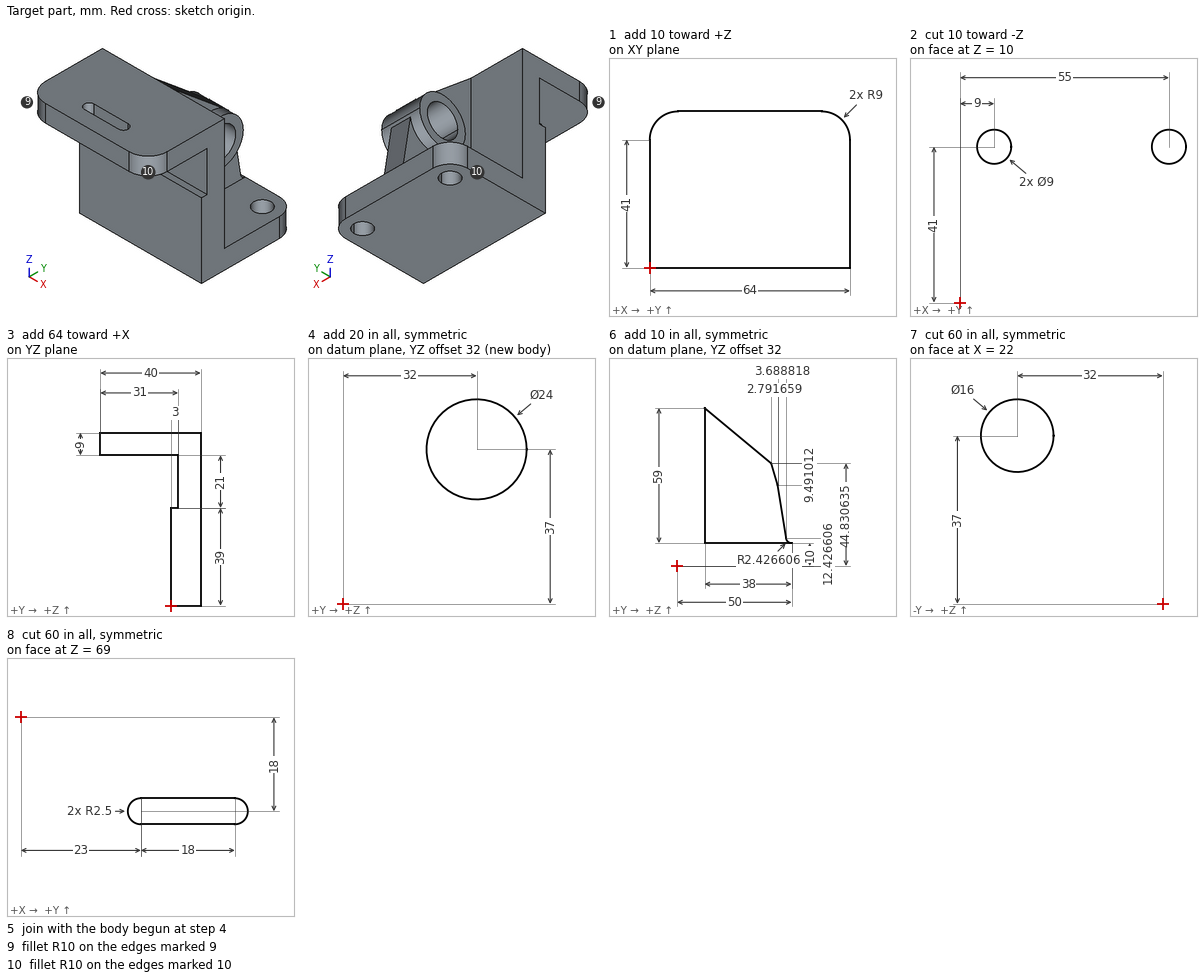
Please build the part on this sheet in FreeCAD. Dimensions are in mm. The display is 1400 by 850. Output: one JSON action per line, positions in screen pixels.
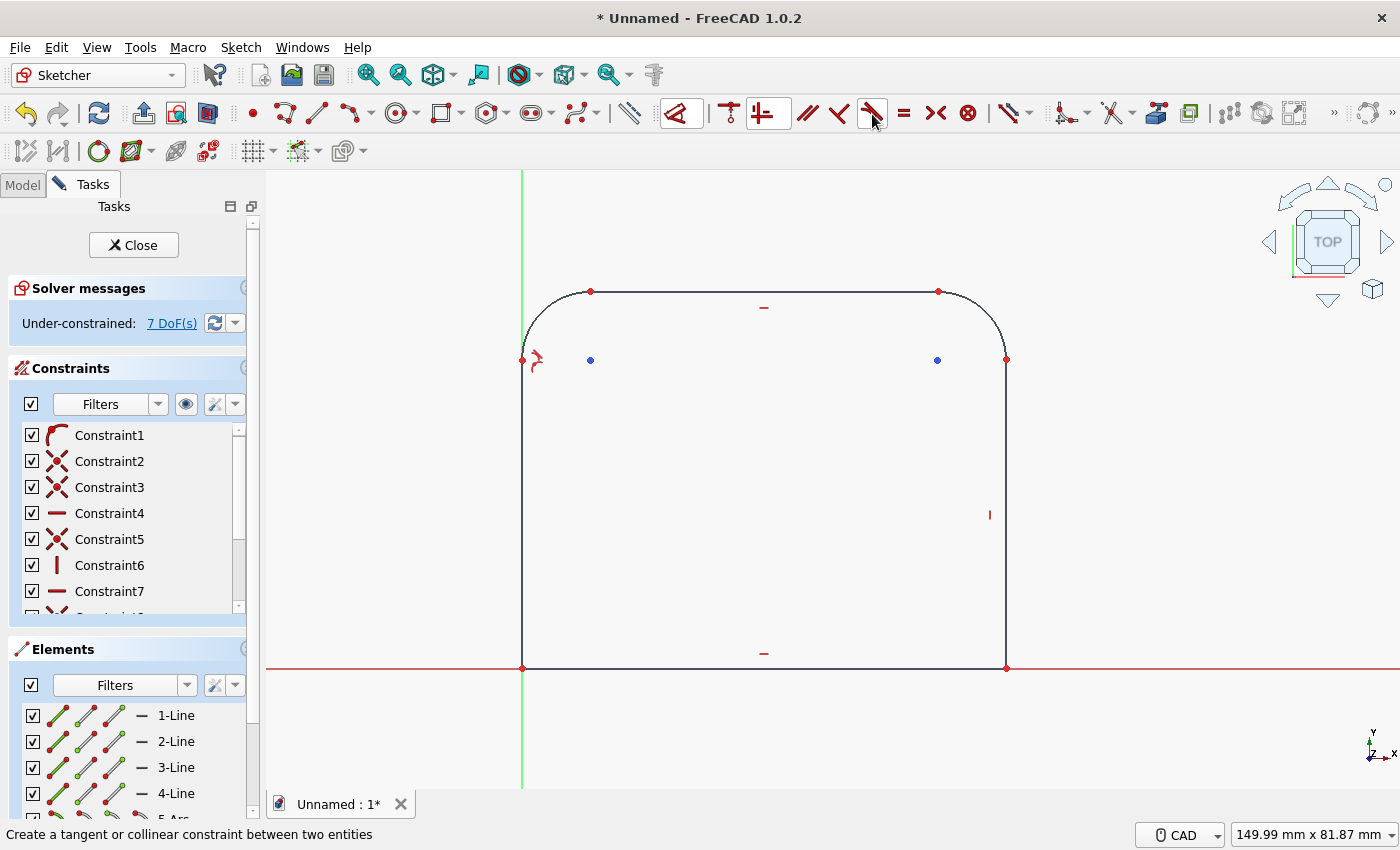
{"action": "left_click", "coordinate": [1006, 576]}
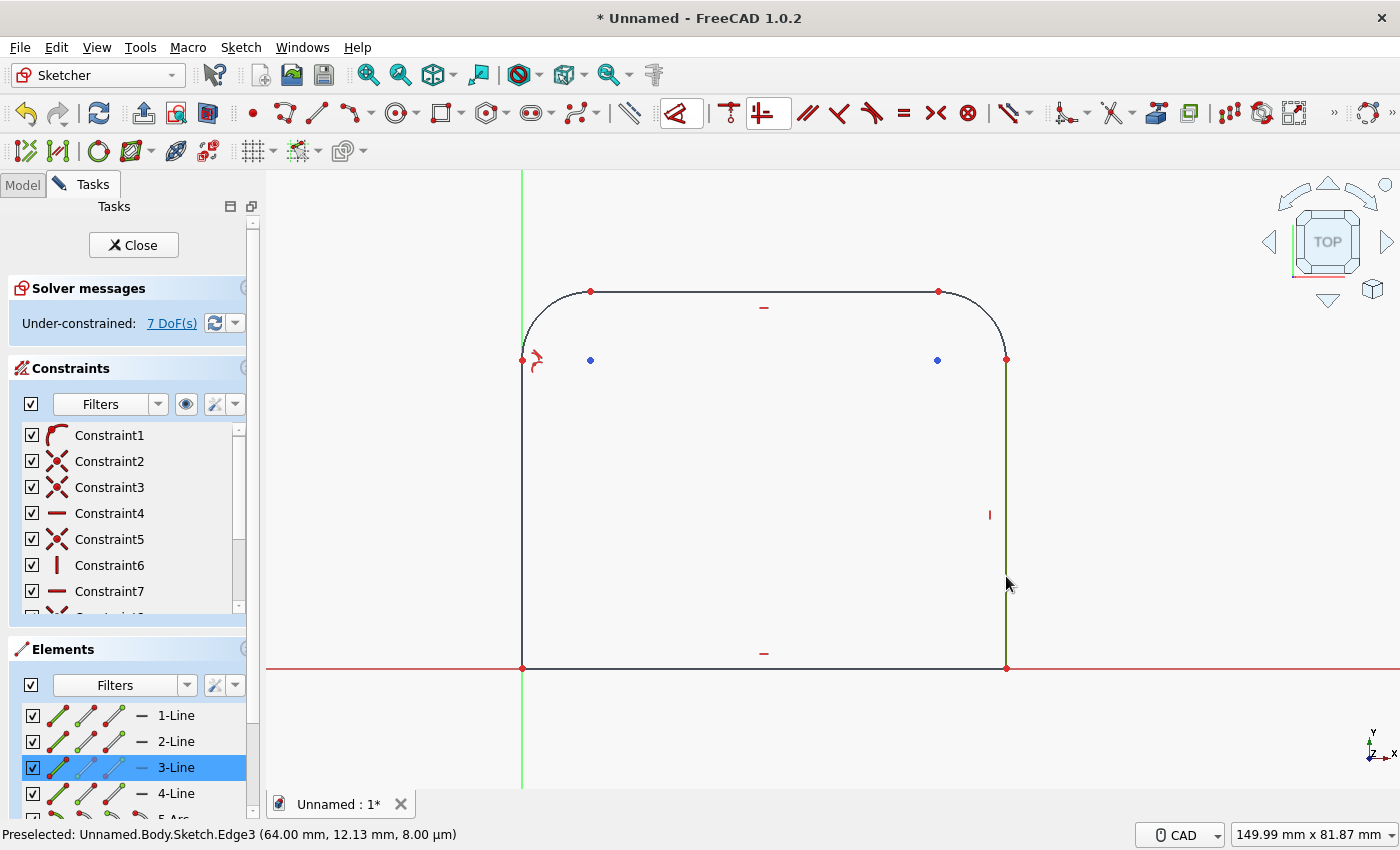
{"action": "left_click", "coordinate": [999, 329]}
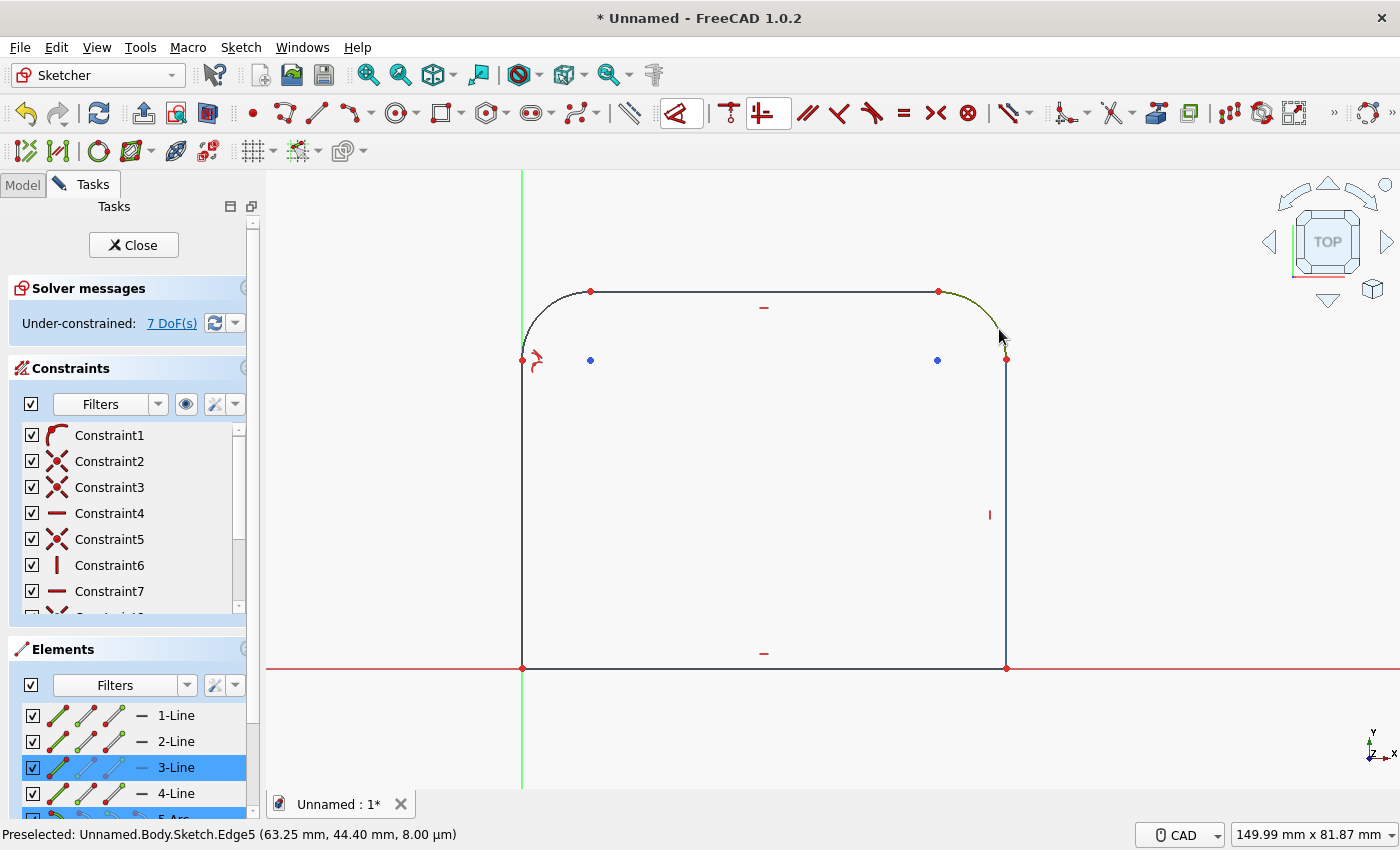
{"action": "left_click", "coordinate": [872, 114]}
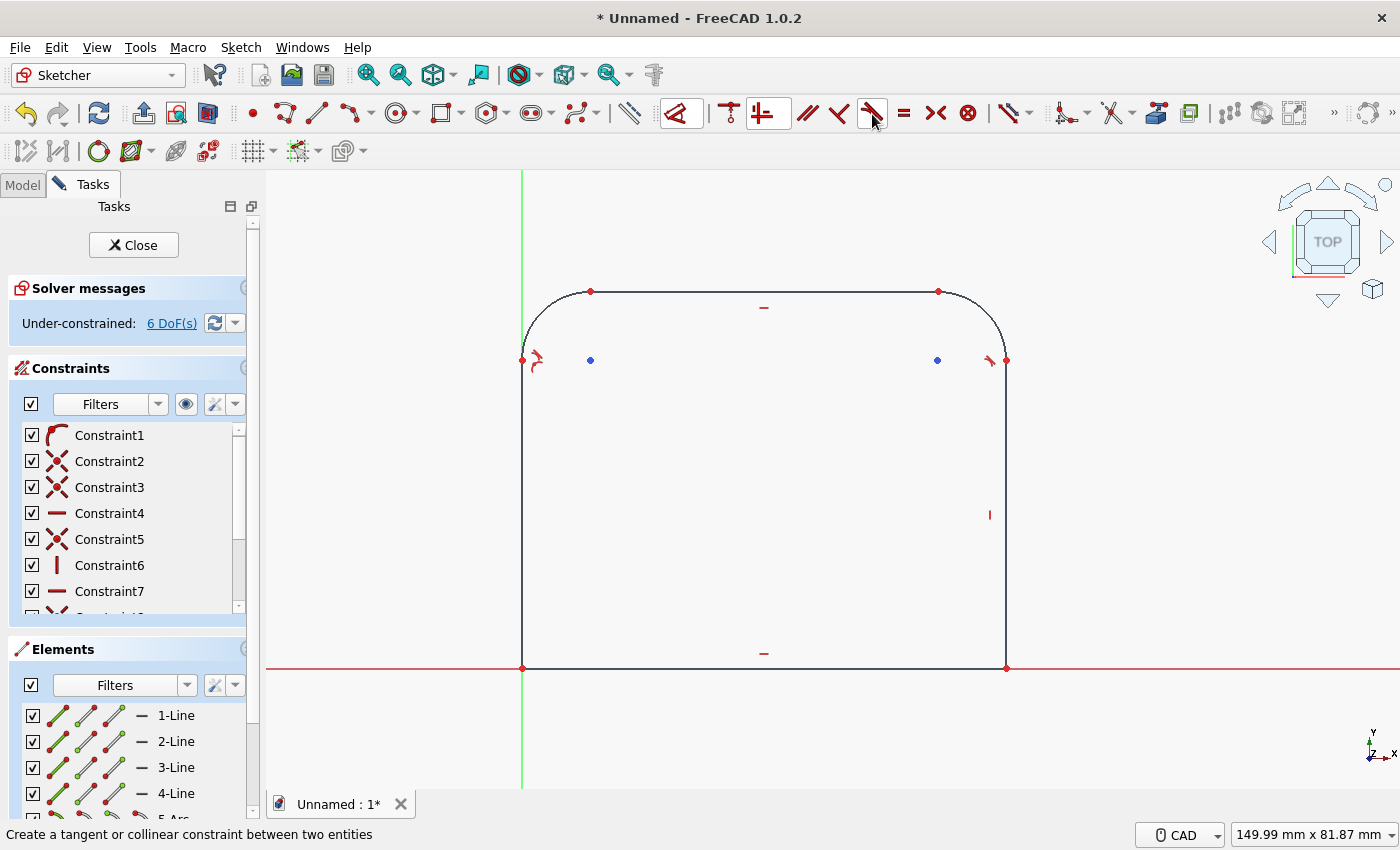
{"action": "left_click", "coordinate": [834, 292]}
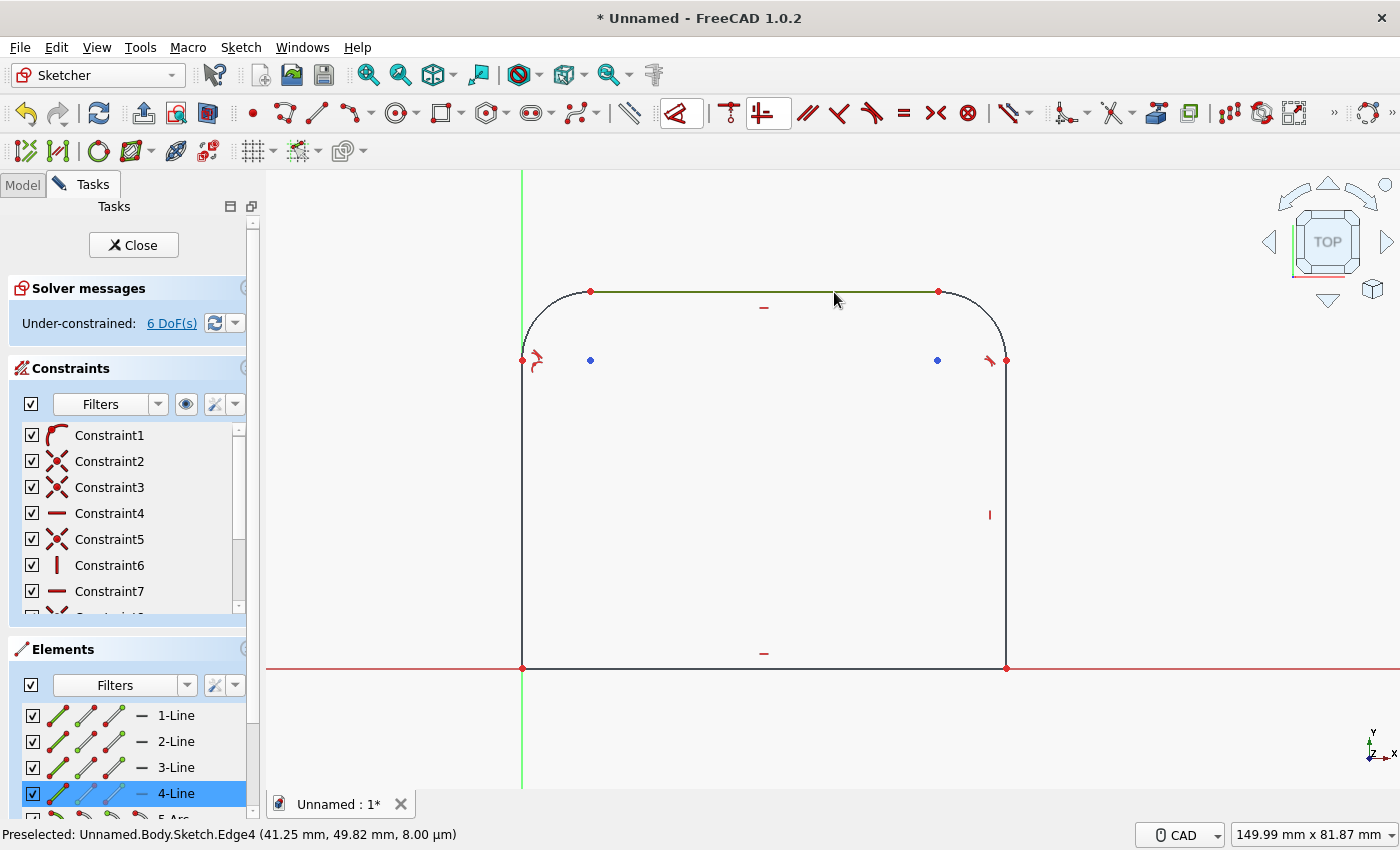
{"action": "left_click", "coordinate": [999, 329]}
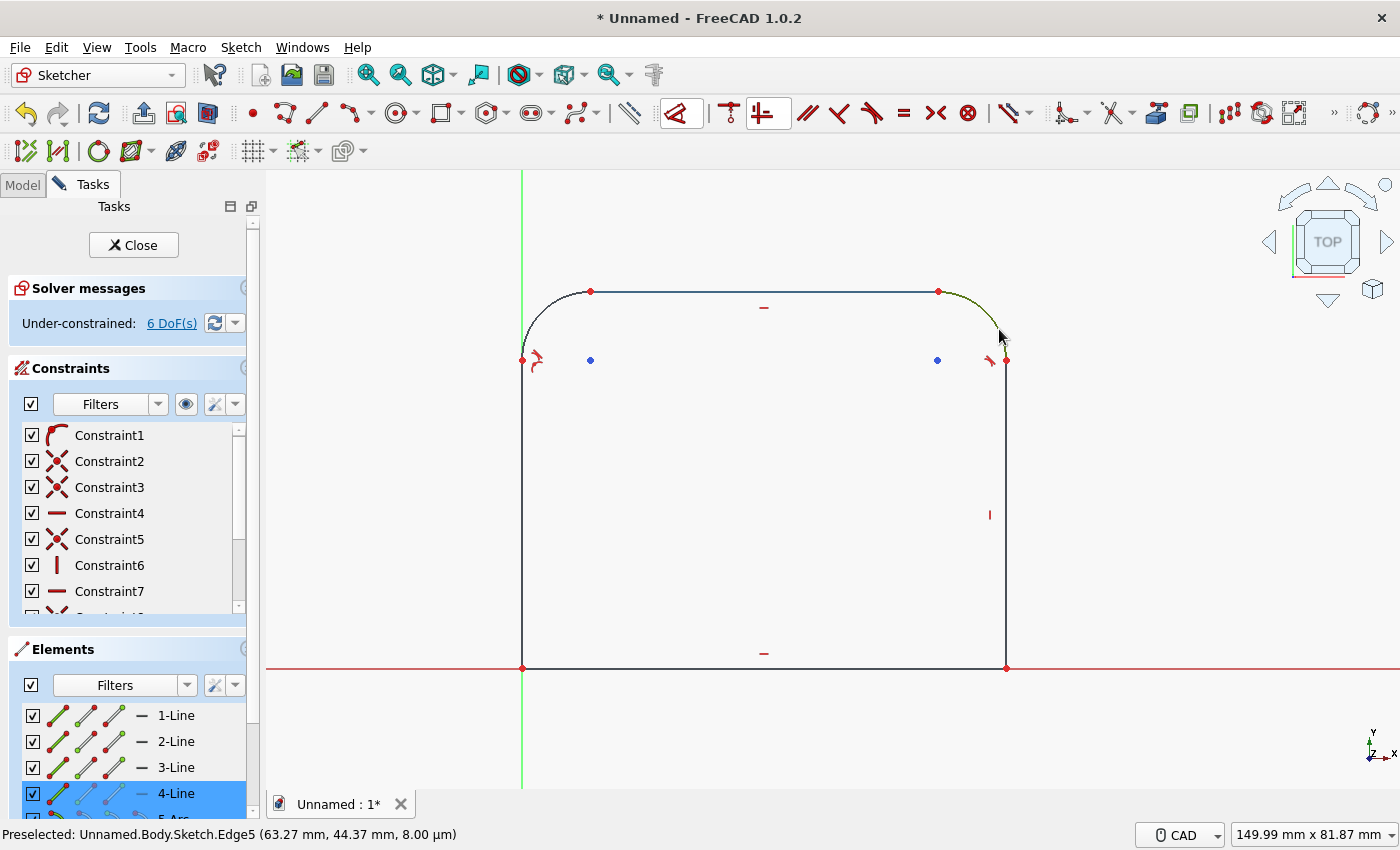
{"action": "left_click", "coordinate": [872, 114]}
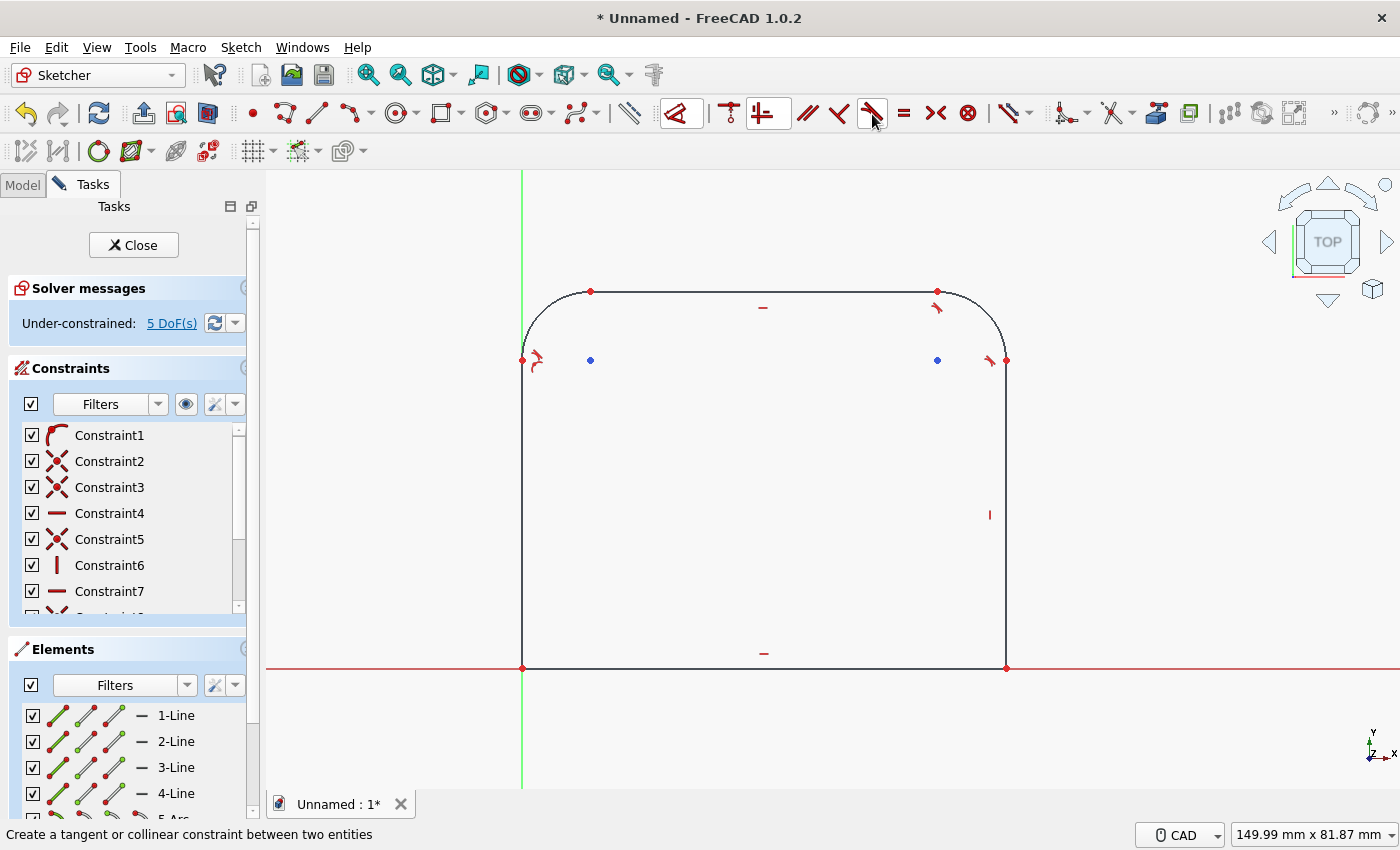
{"action": "left_click", "coordinate": [833, 292]}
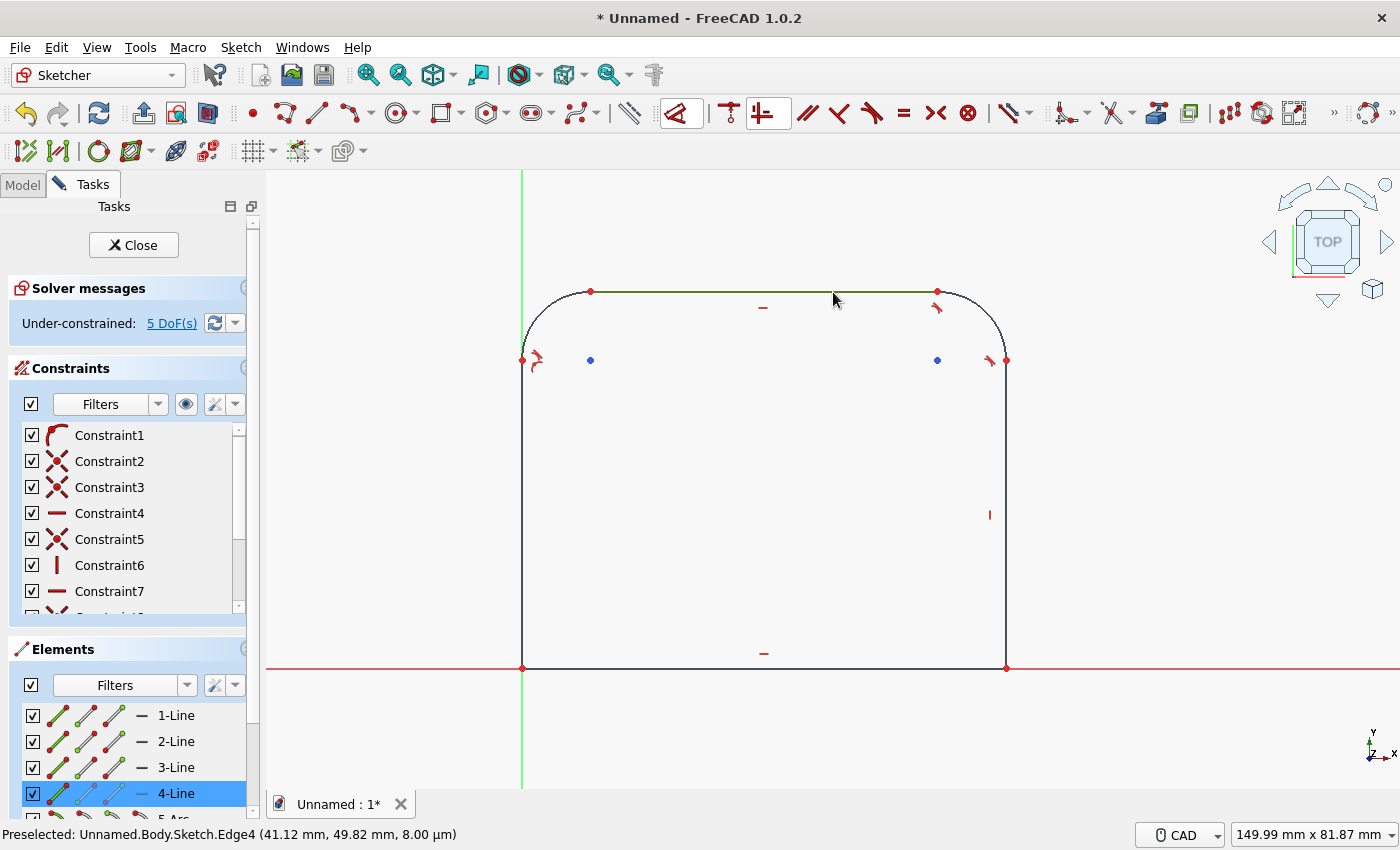
{"action": "left_click", "coordinate": [559, 299]}